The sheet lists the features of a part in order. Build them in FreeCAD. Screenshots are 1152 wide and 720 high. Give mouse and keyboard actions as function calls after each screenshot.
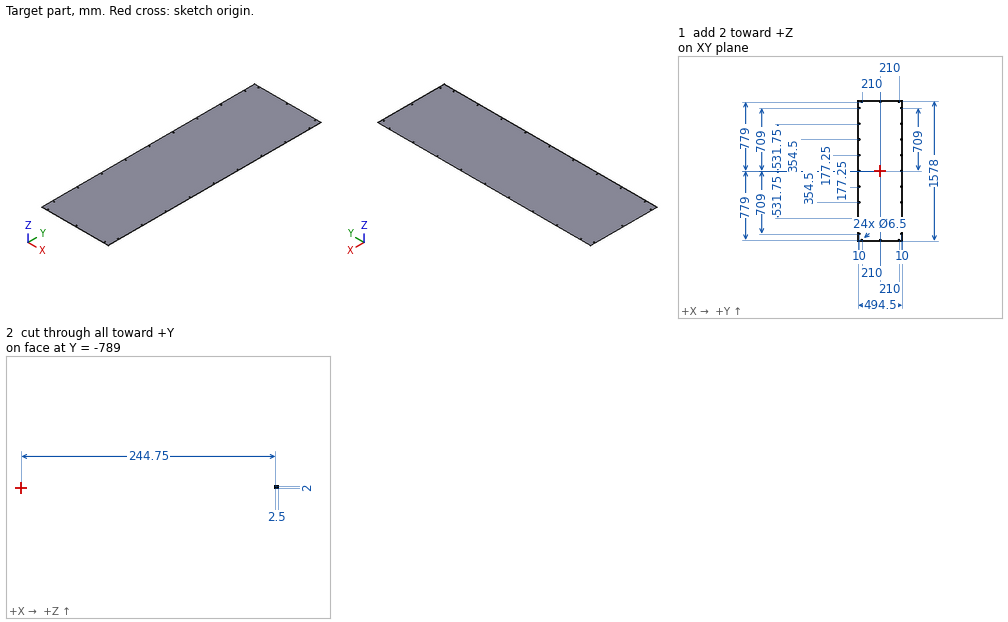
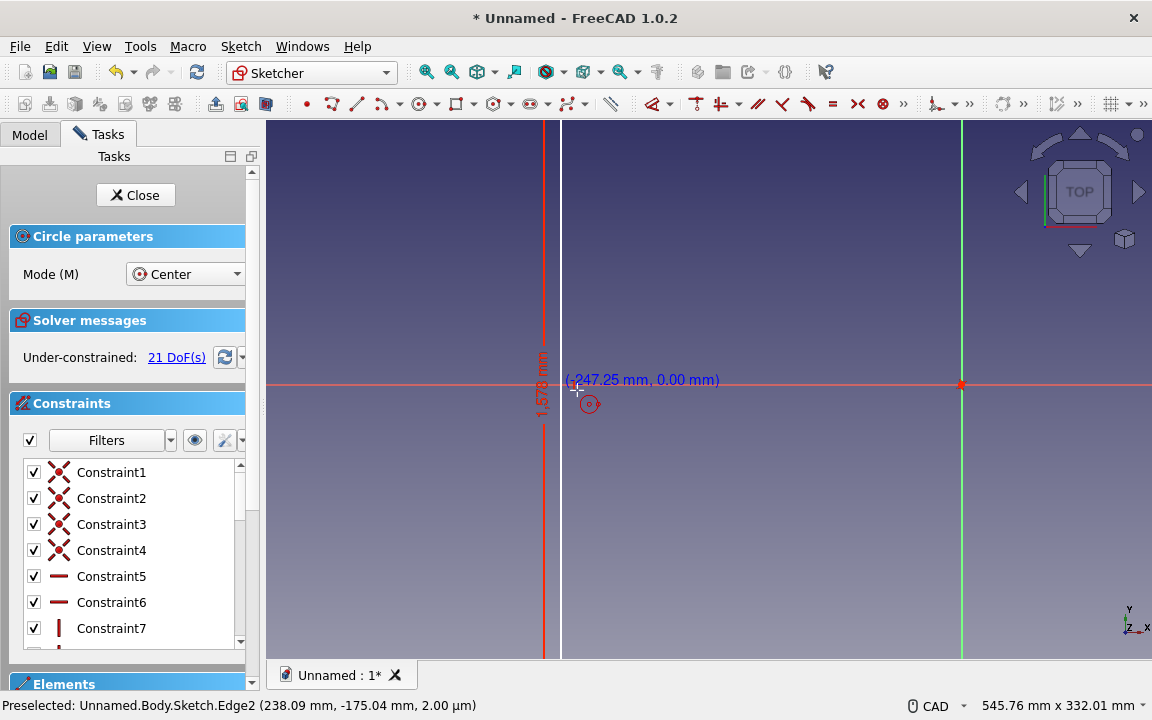
click(577, 385)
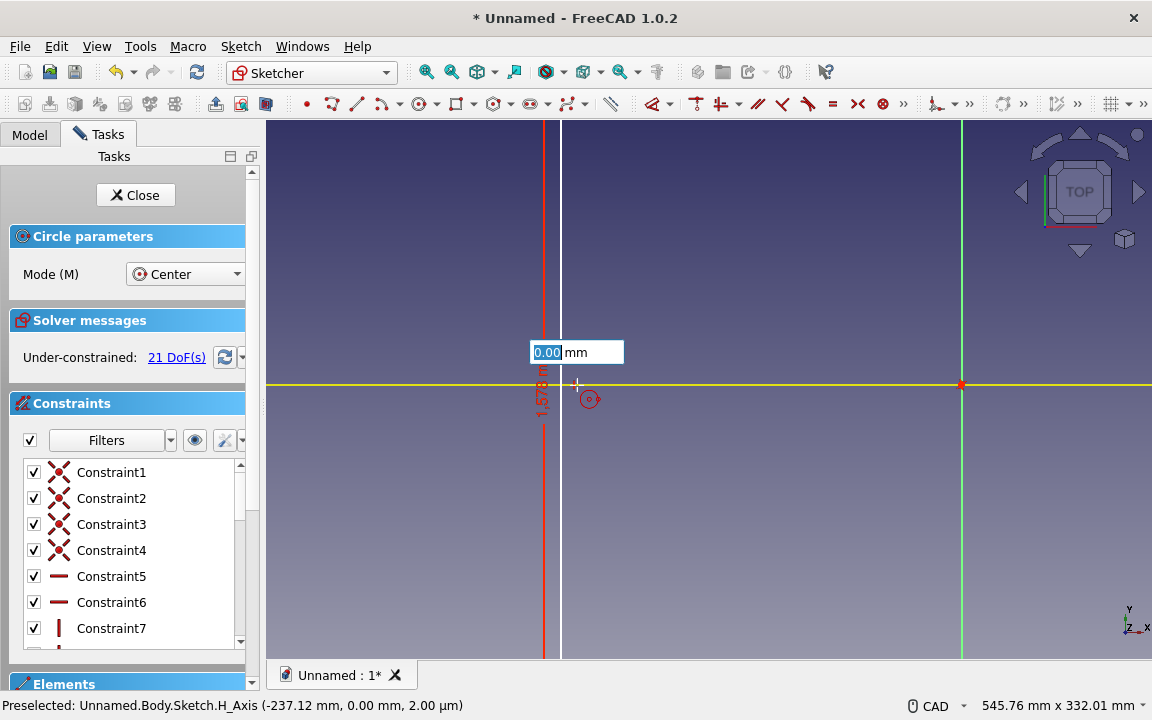
scroll(579, 380, up, 6)
move(577, 378)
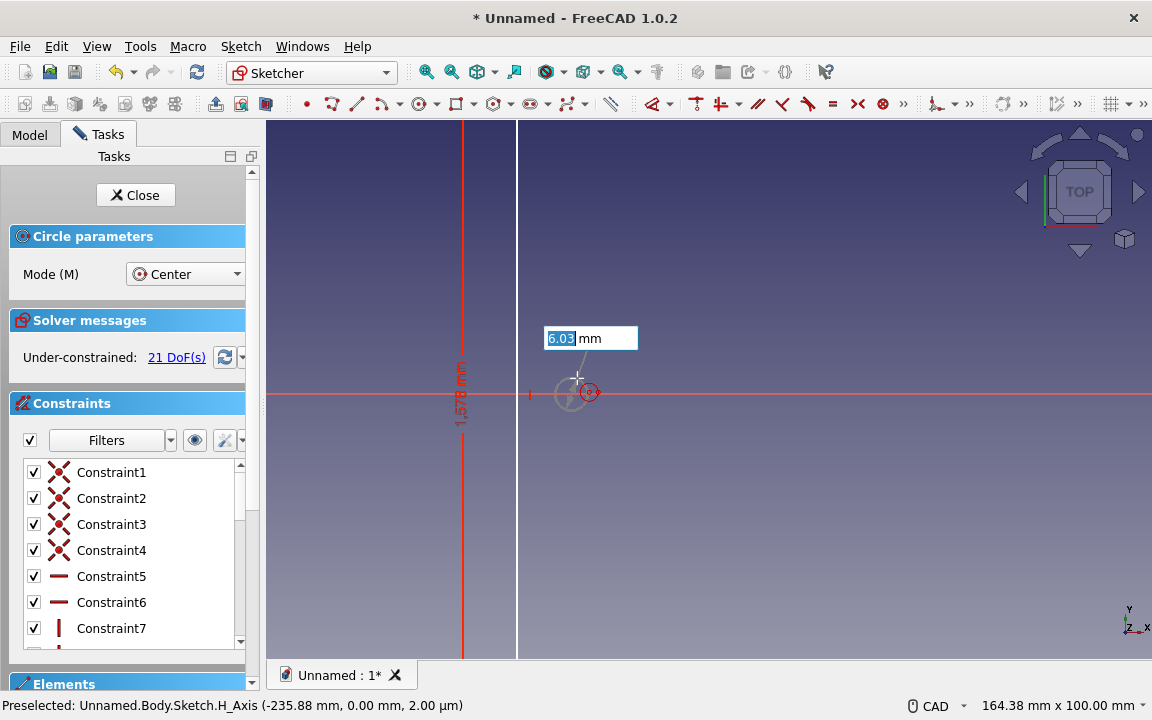
text(6.5)
key(Return)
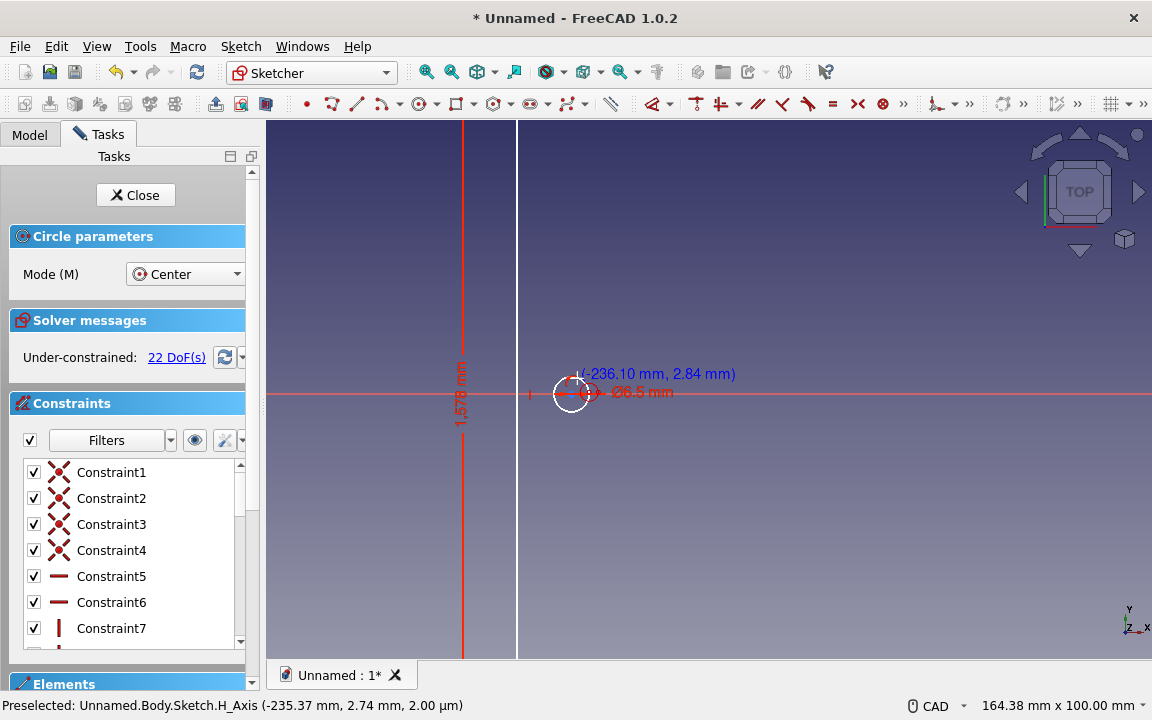
scroll(577, 389, down, 15)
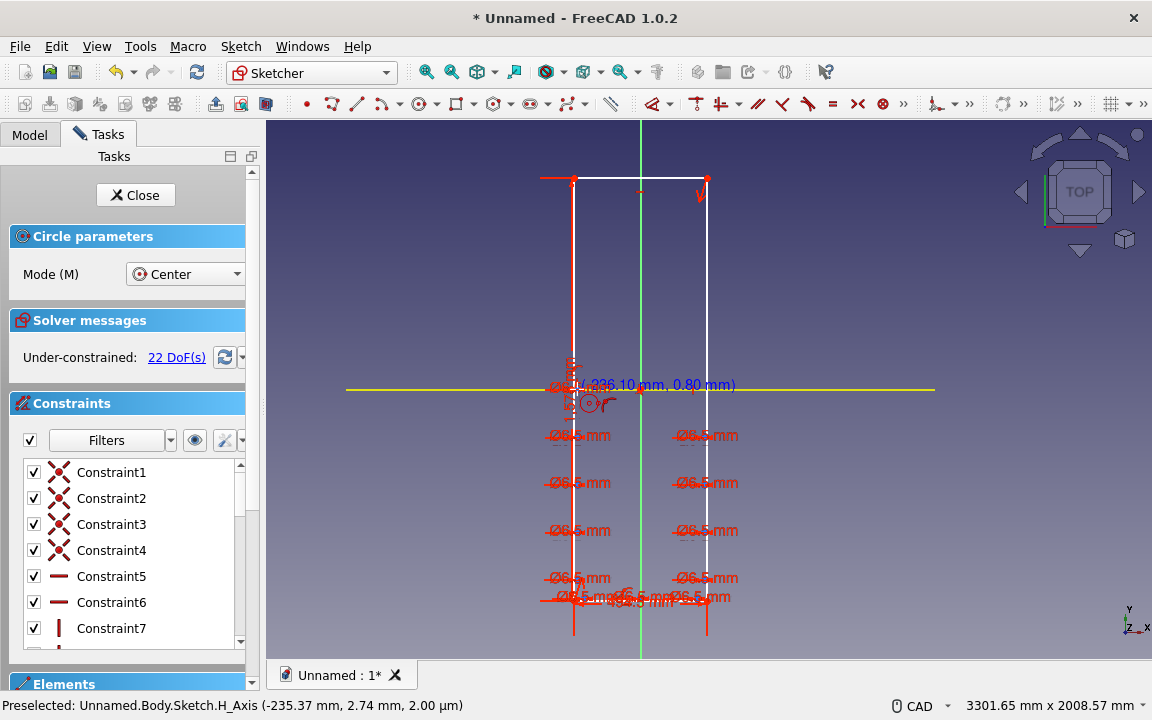
scroll(577, 342, up, 17)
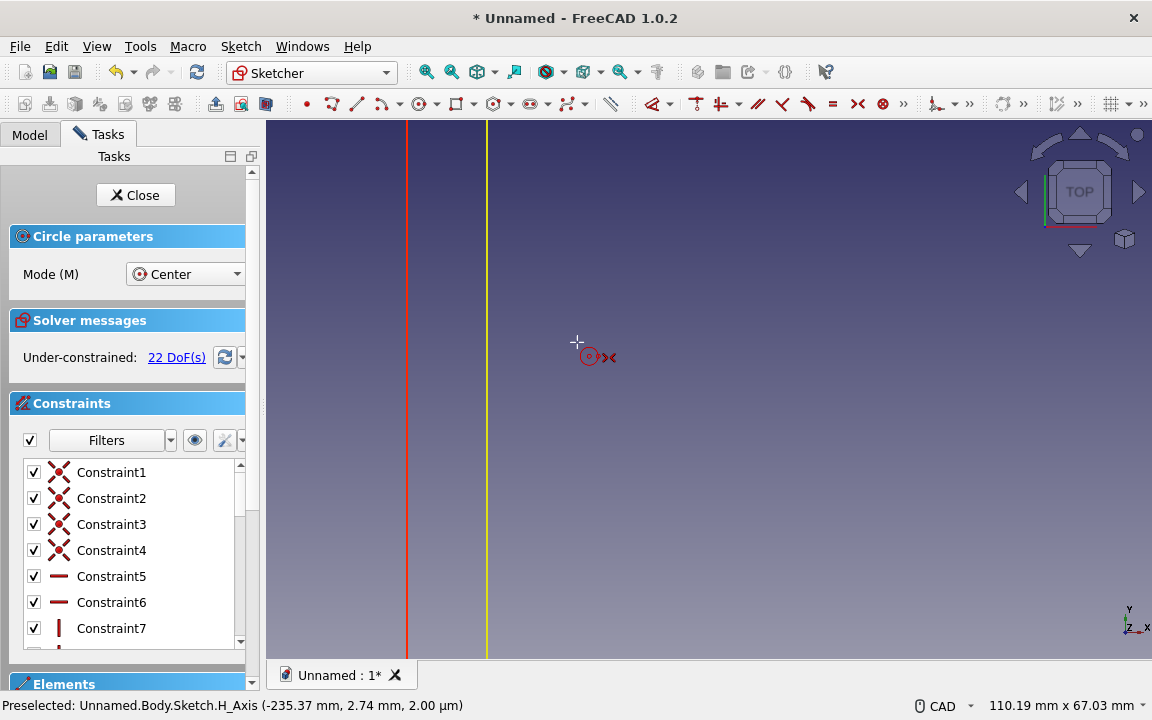
scroll(577, 342, down, 17)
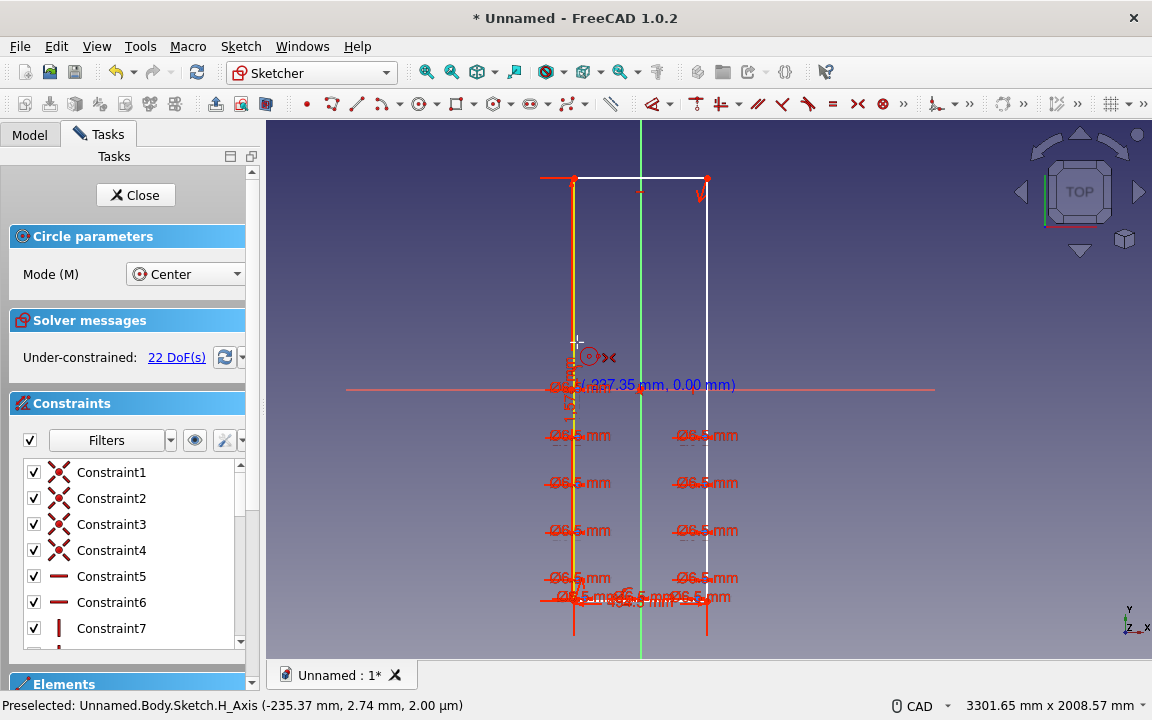
scroll(577, 342, up, 9)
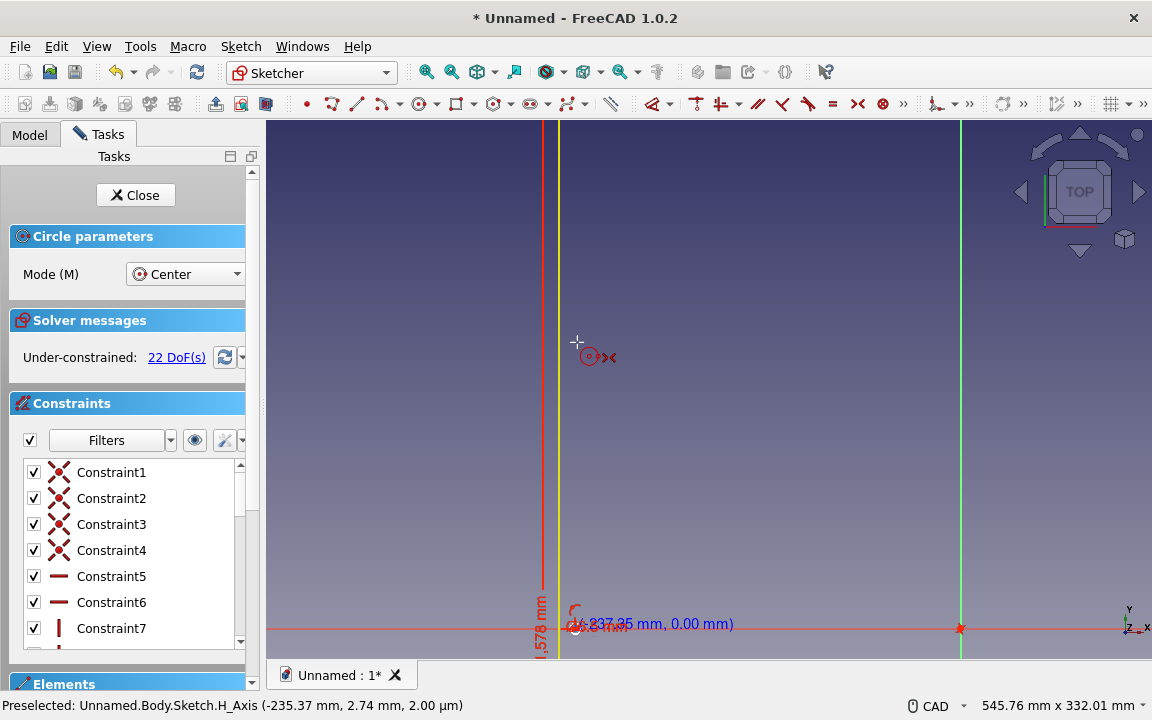
click(575, 341)
move(579, 337)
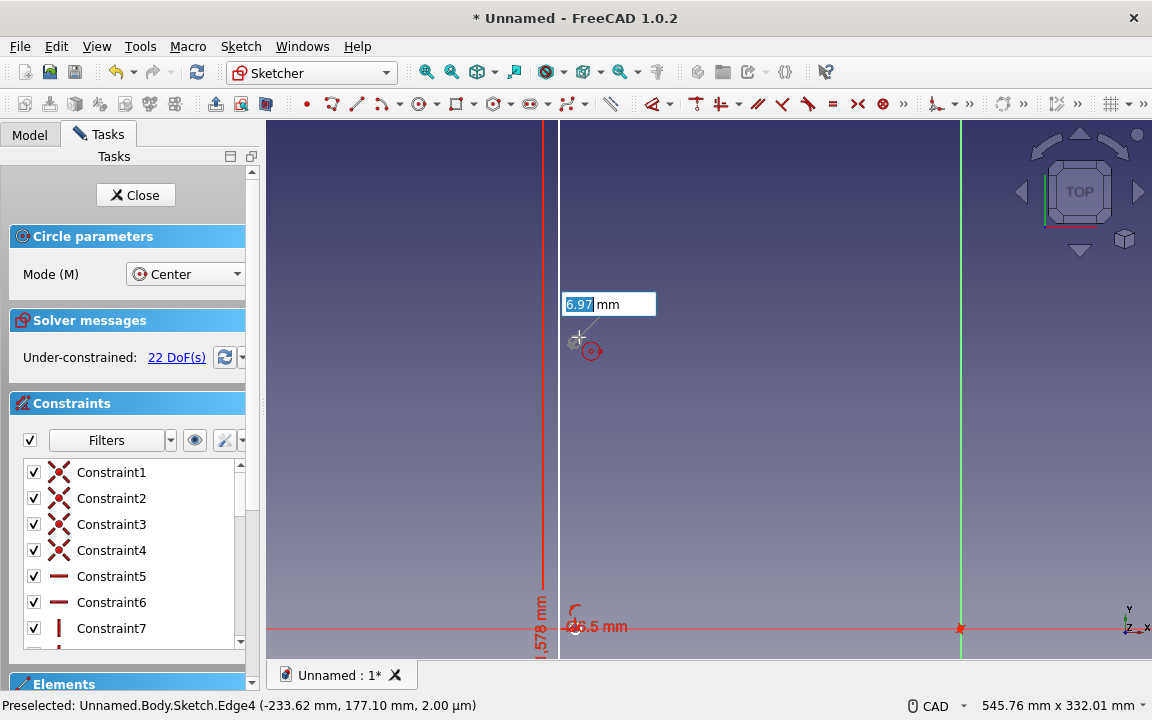
text(6.5)
key(Return)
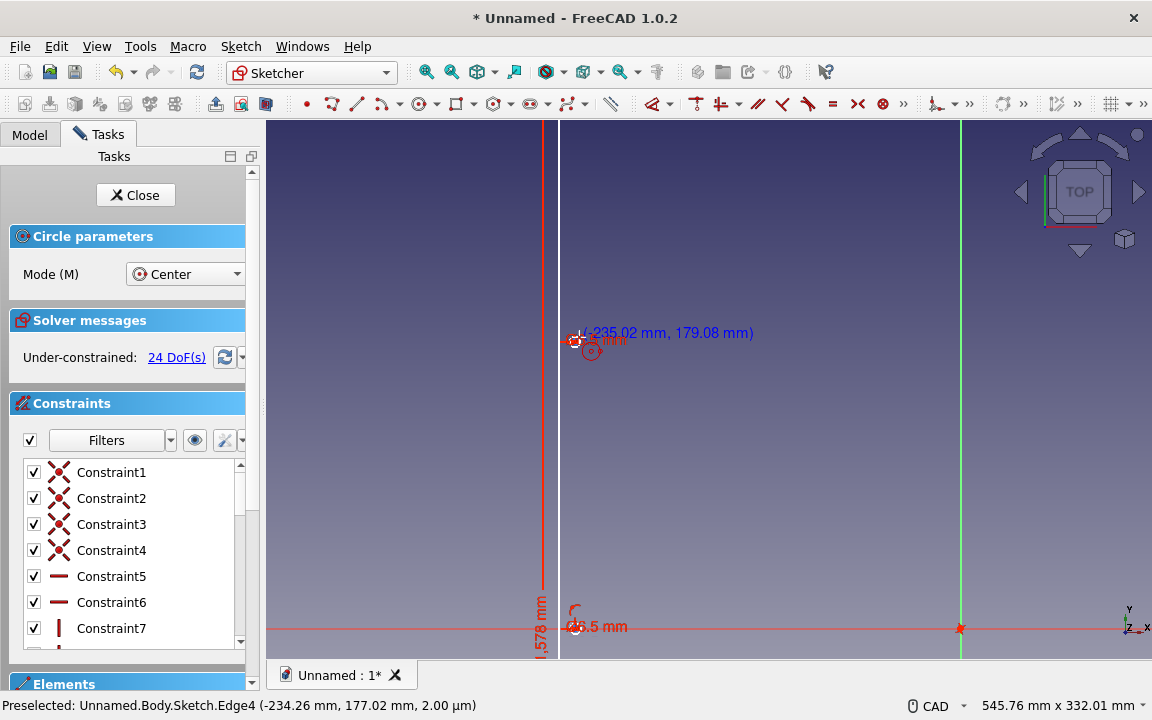
scroll(590, 352, down, 10)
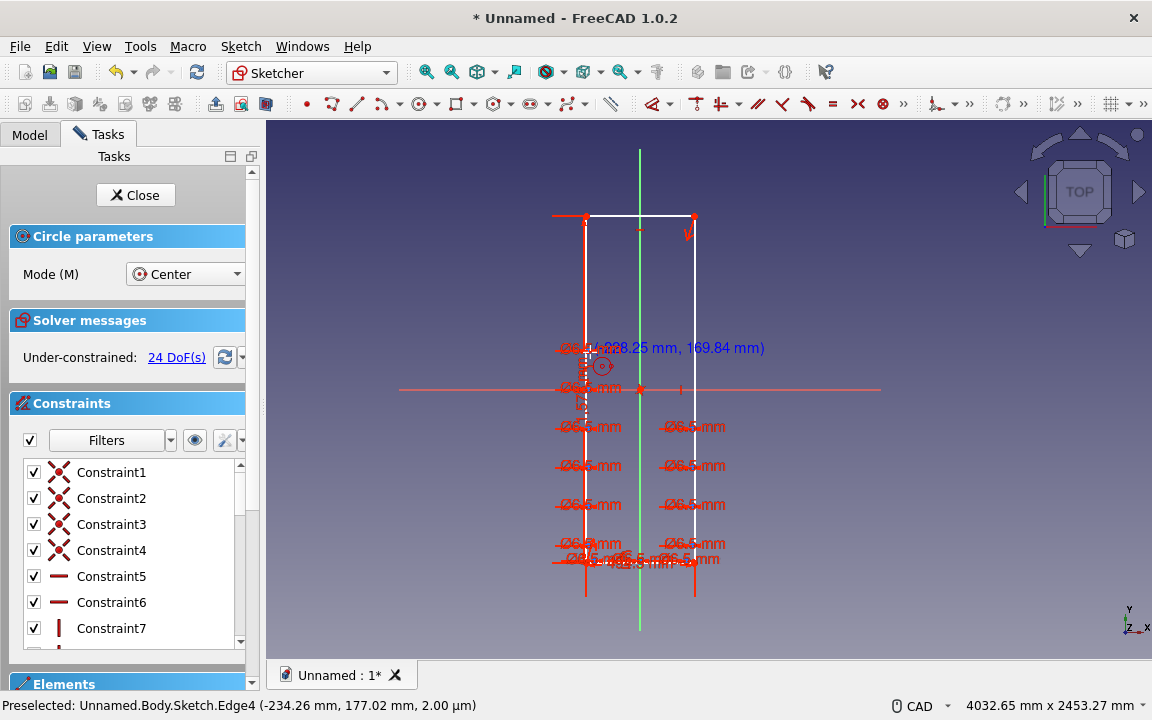
scroll(588, 312, up, 18)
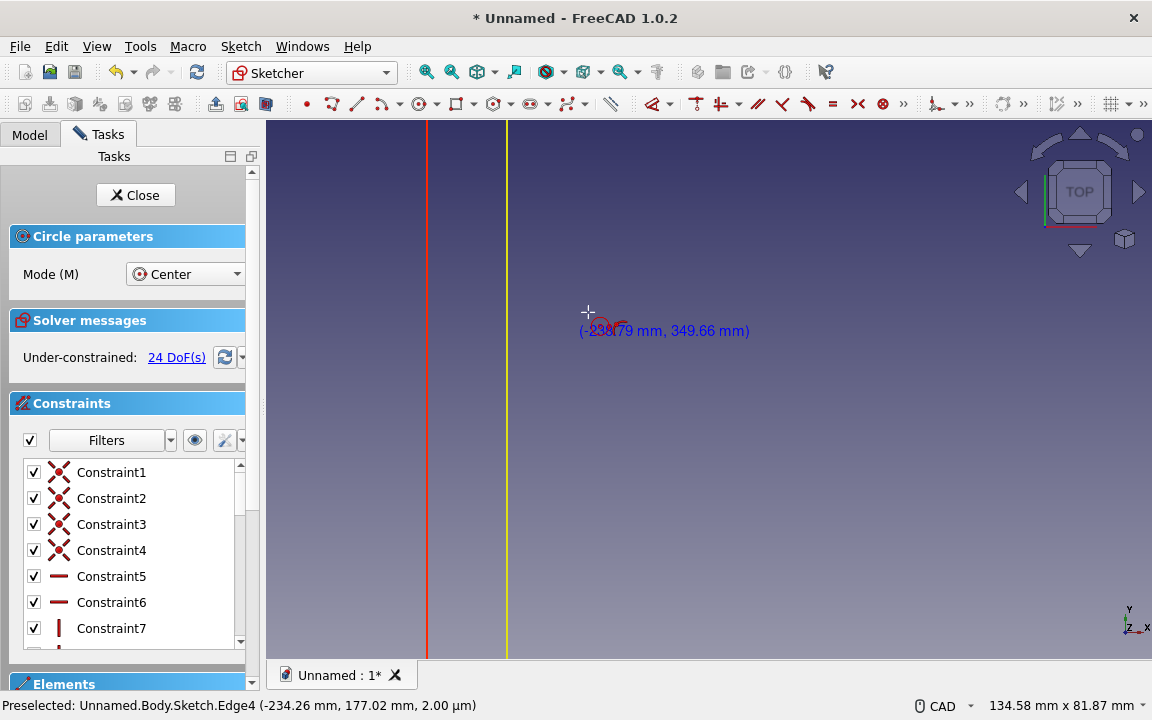
scroll(576, 294, down, 17)